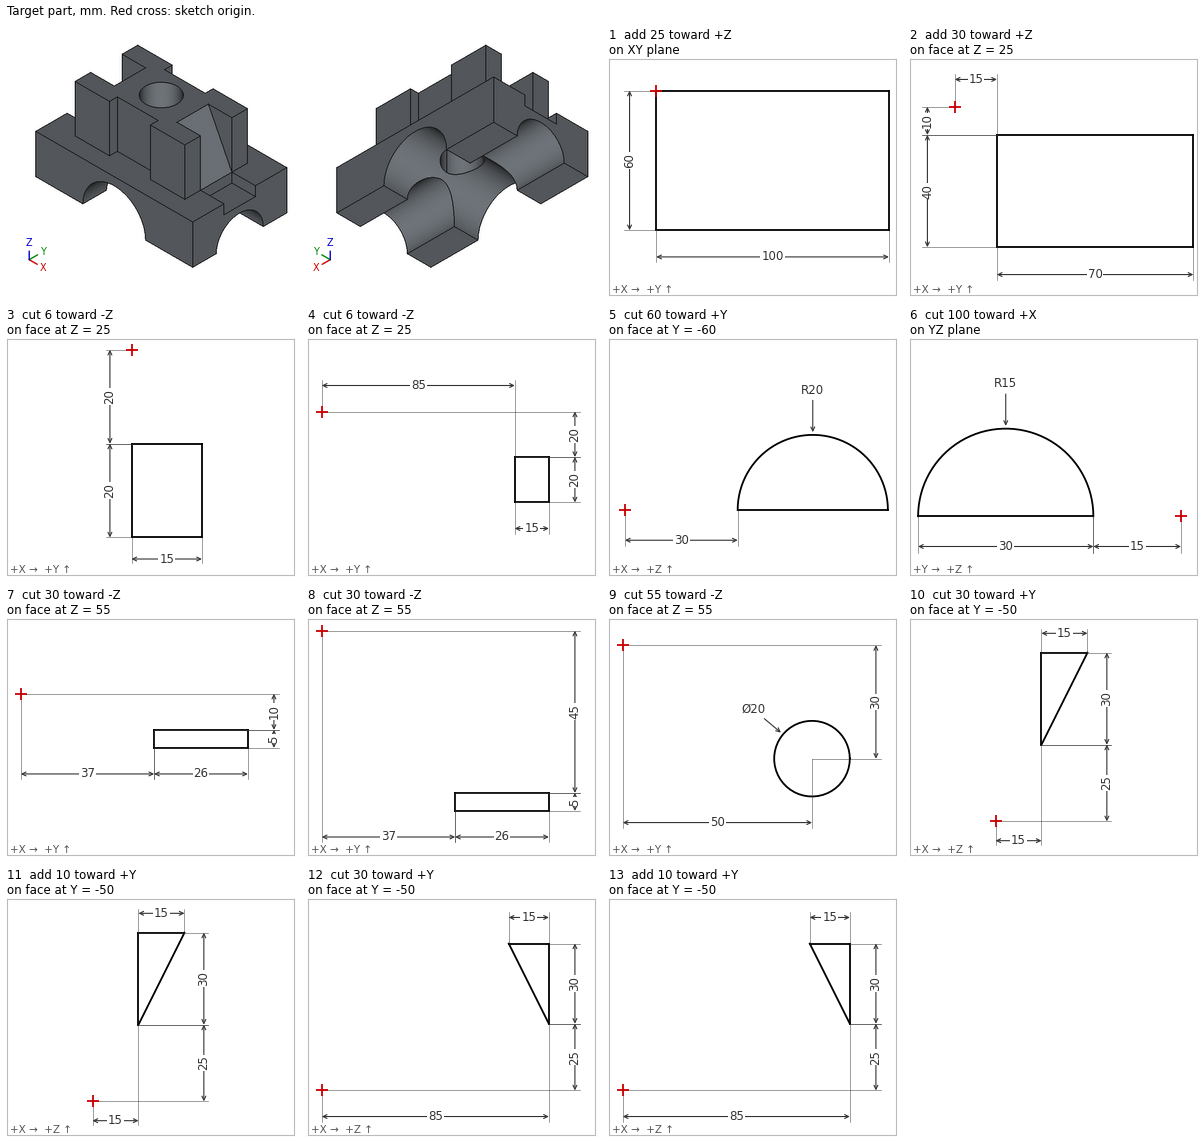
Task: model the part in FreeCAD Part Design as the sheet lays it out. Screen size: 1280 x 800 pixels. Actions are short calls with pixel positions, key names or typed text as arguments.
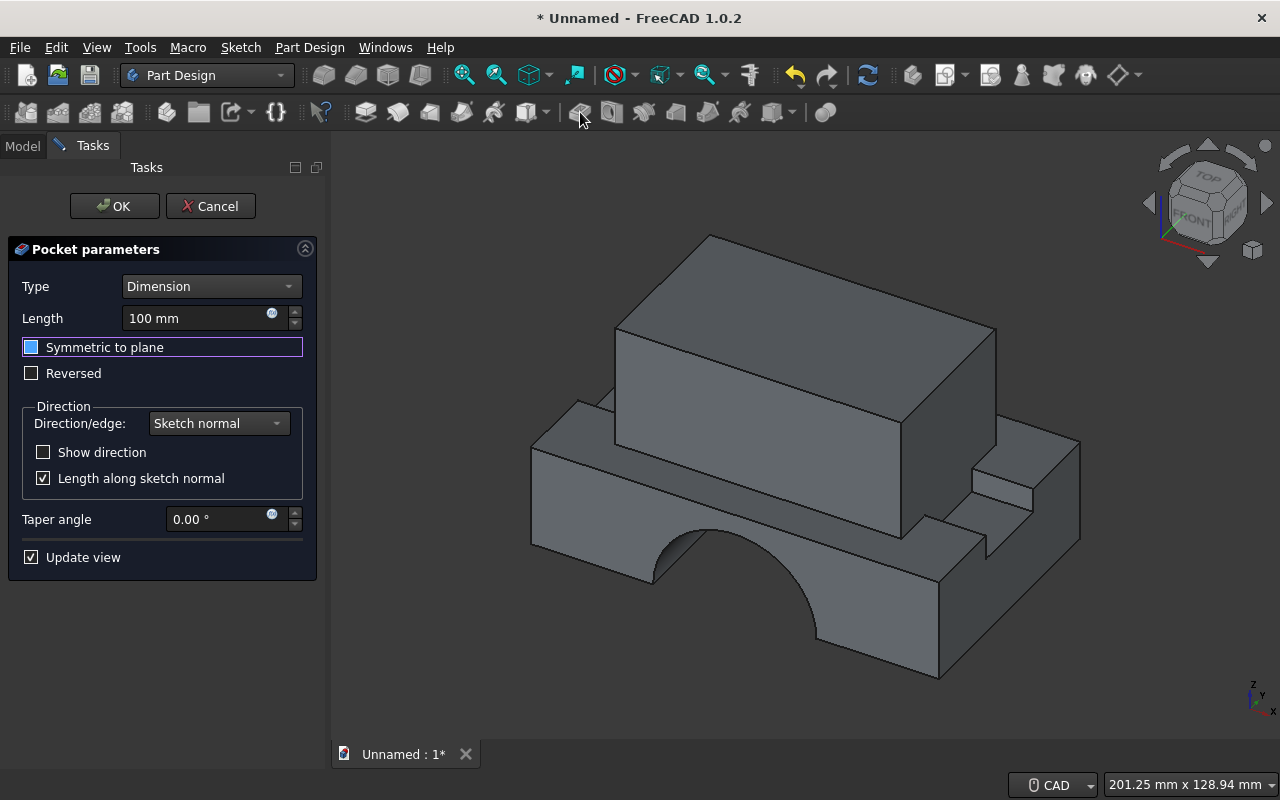
click(30, 373)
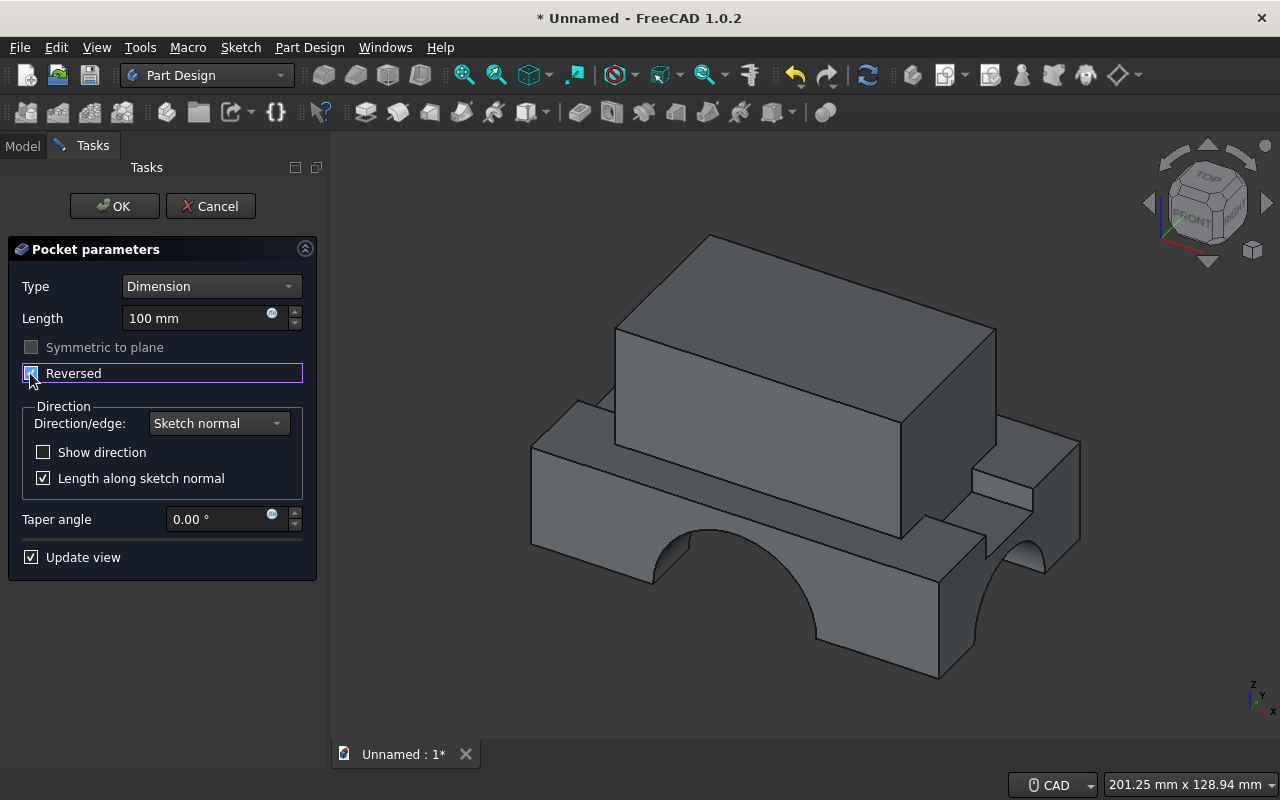
click(115, 206)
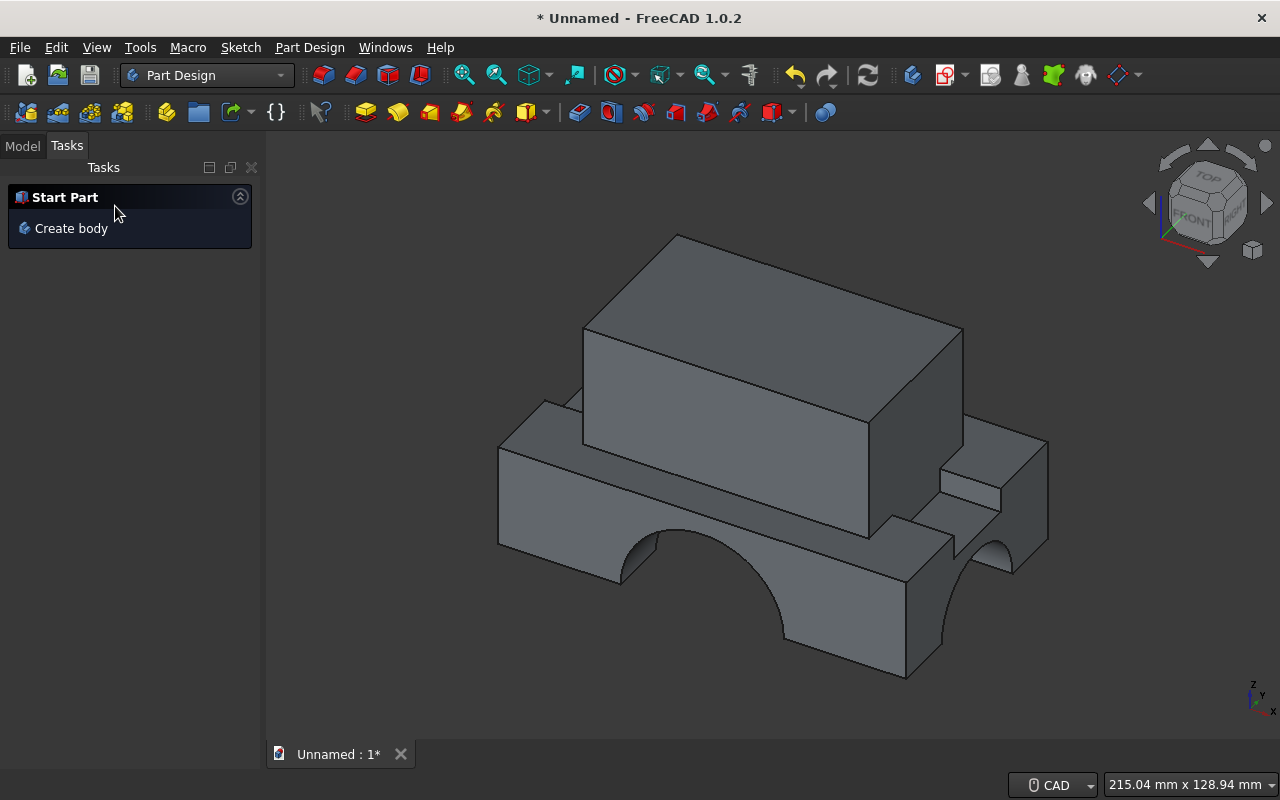
click(814, 341)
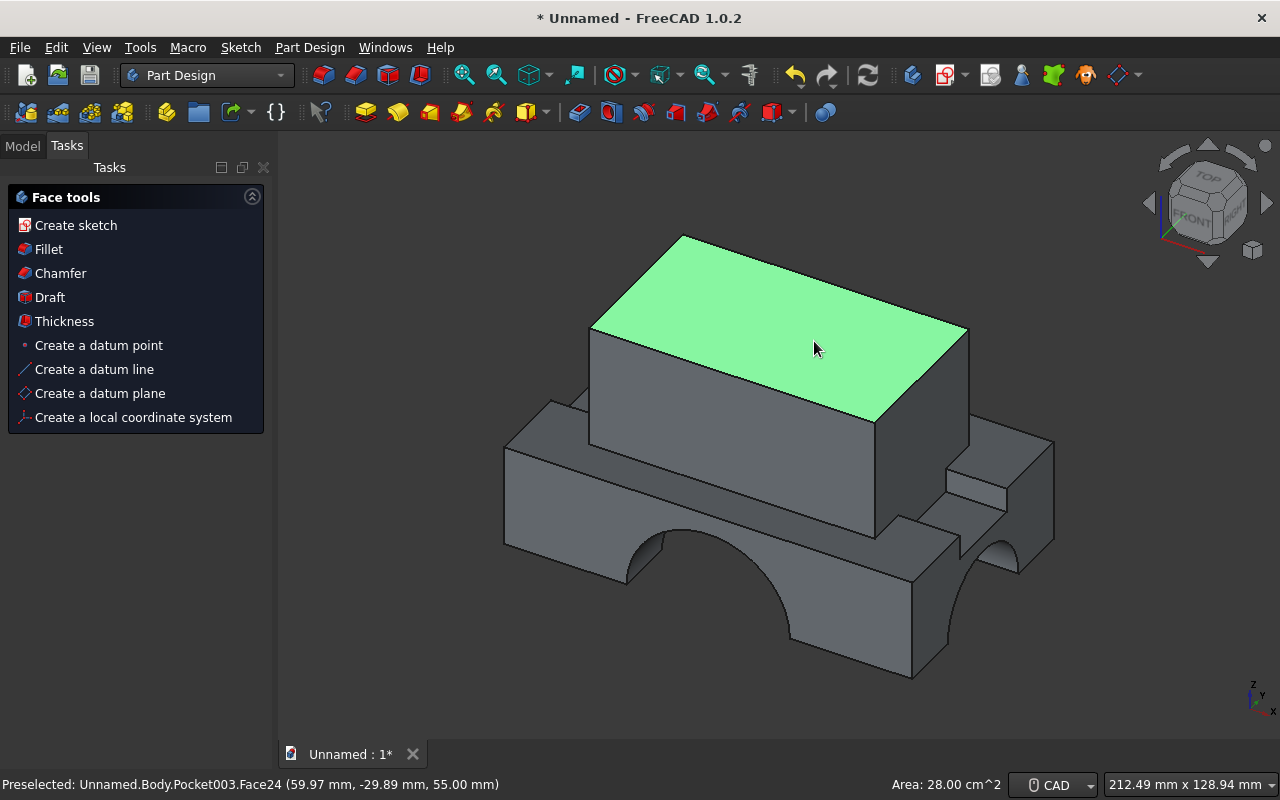
click(946, 76)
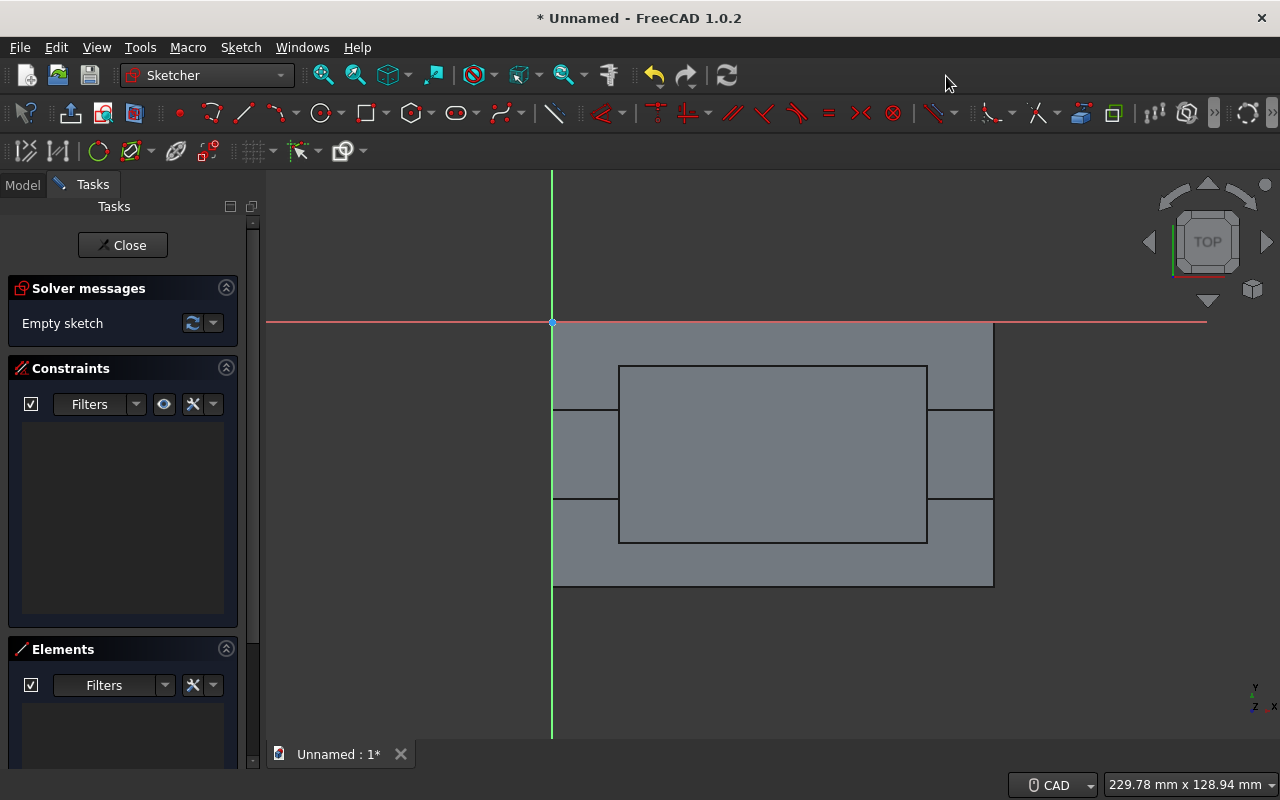
scroll(681, 274, up, 4)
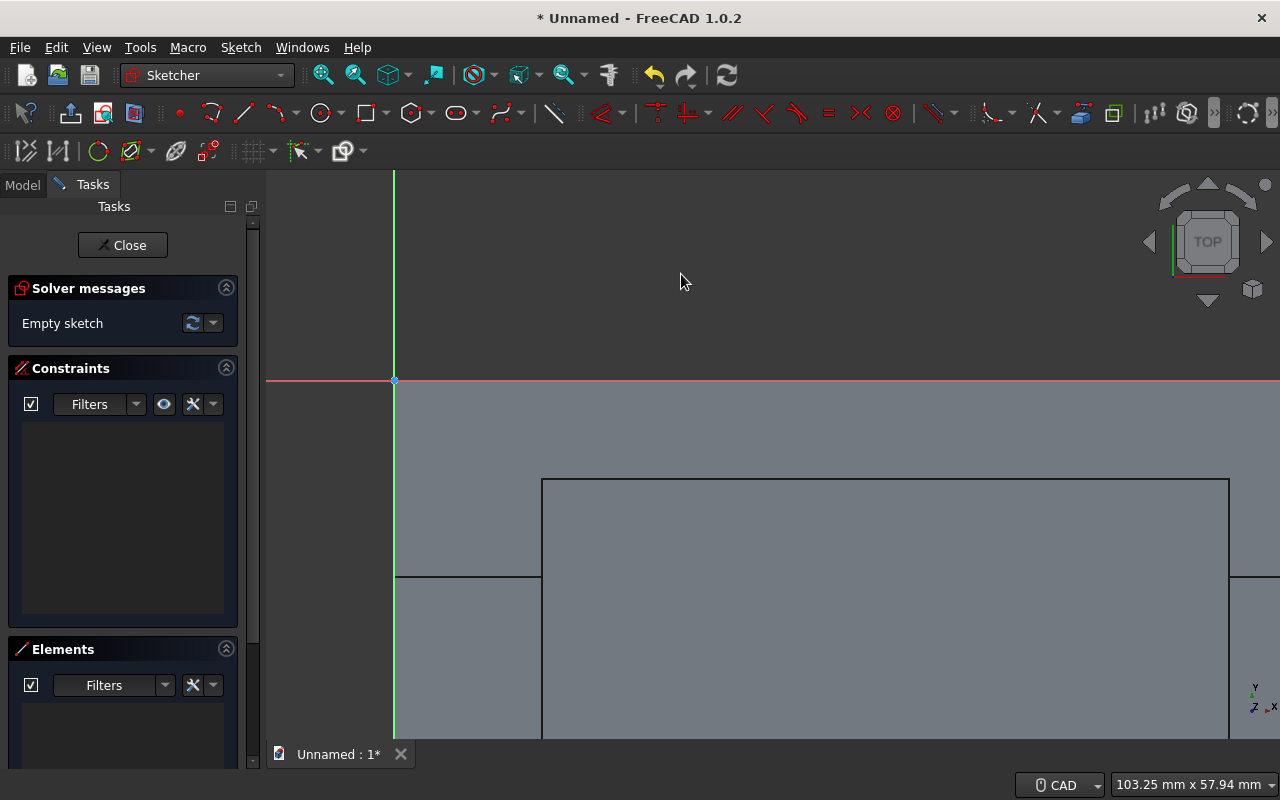
key(g)
key(r)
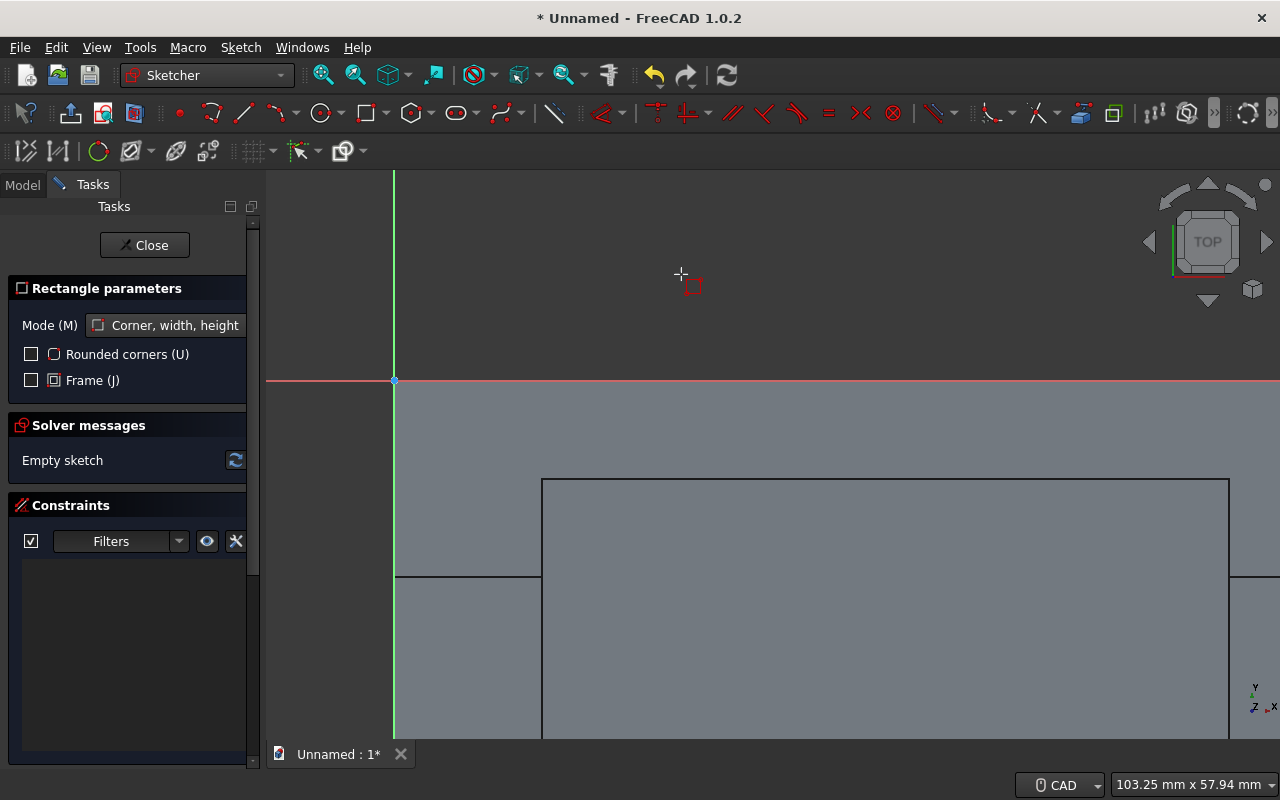
click(758, 479)
click(1013, 528)
key(Escape)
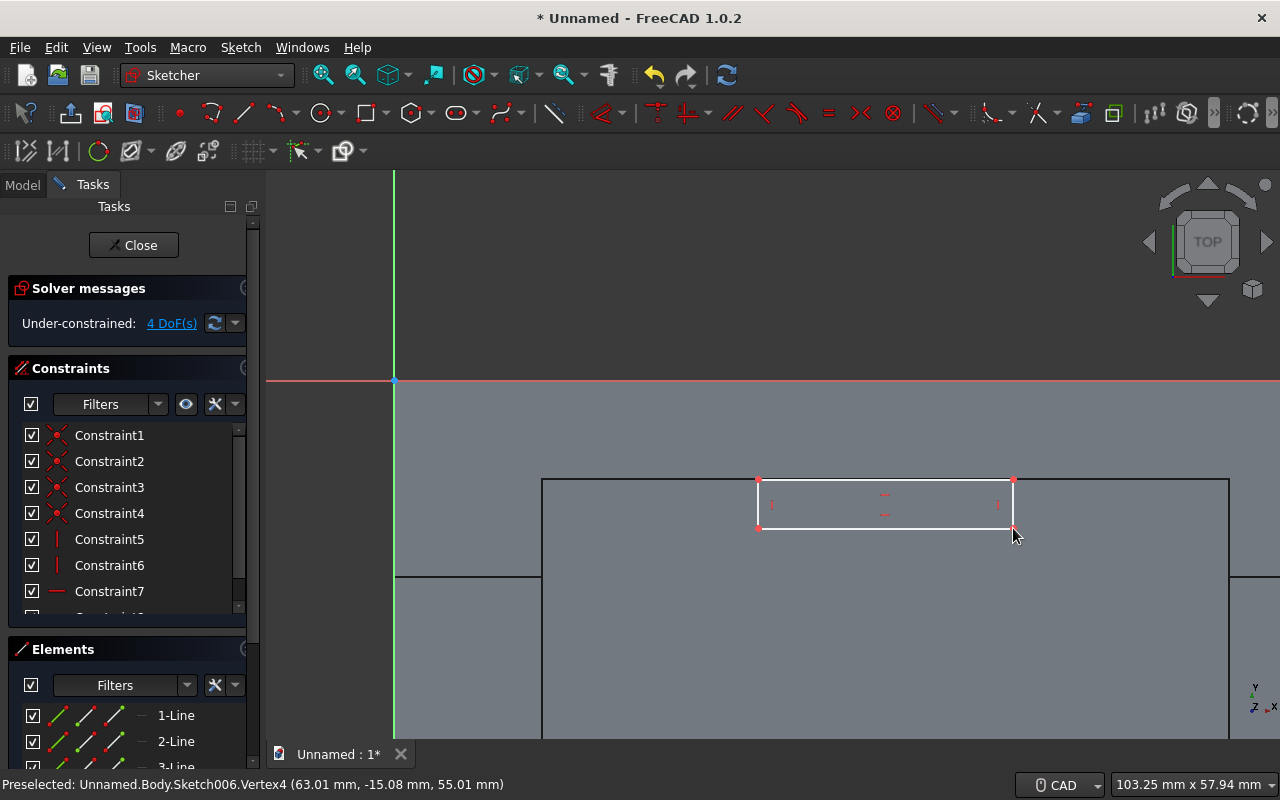
key(d)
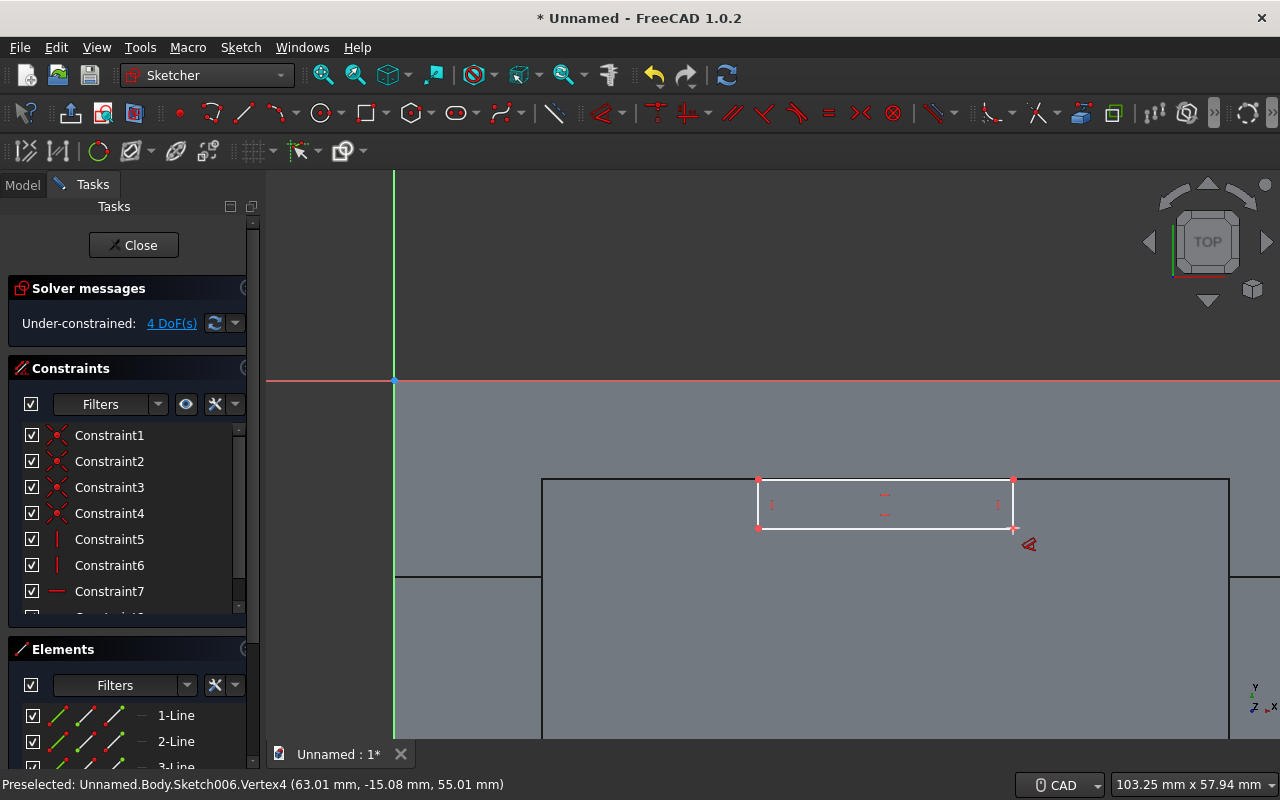
click(758, 495)
click(792, 504)